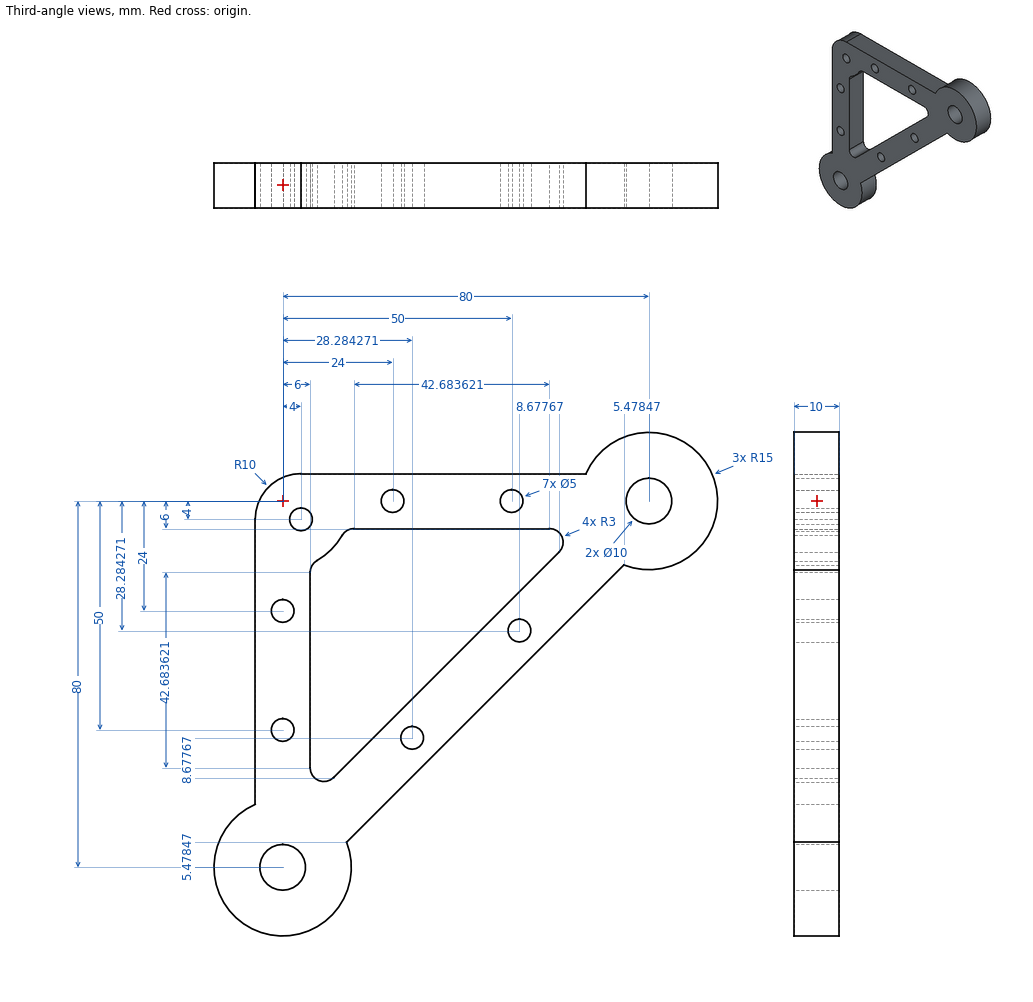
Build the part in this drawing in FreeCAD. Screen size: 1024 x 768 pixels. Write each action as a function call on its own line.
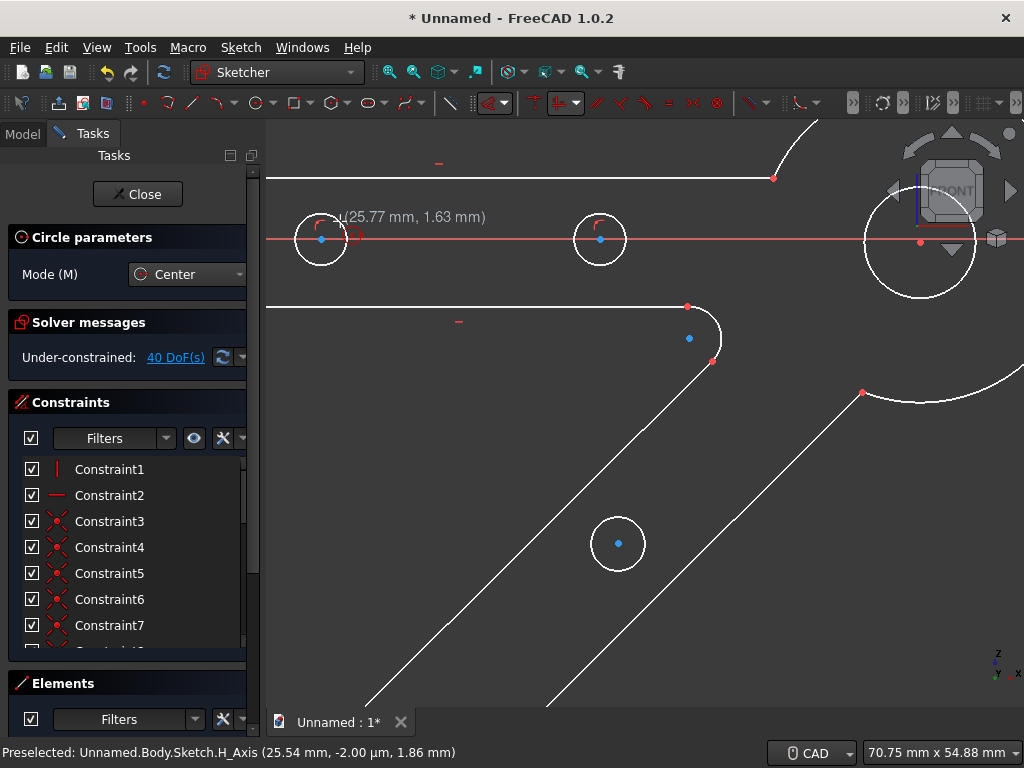
scroll(601, 240, down, 5)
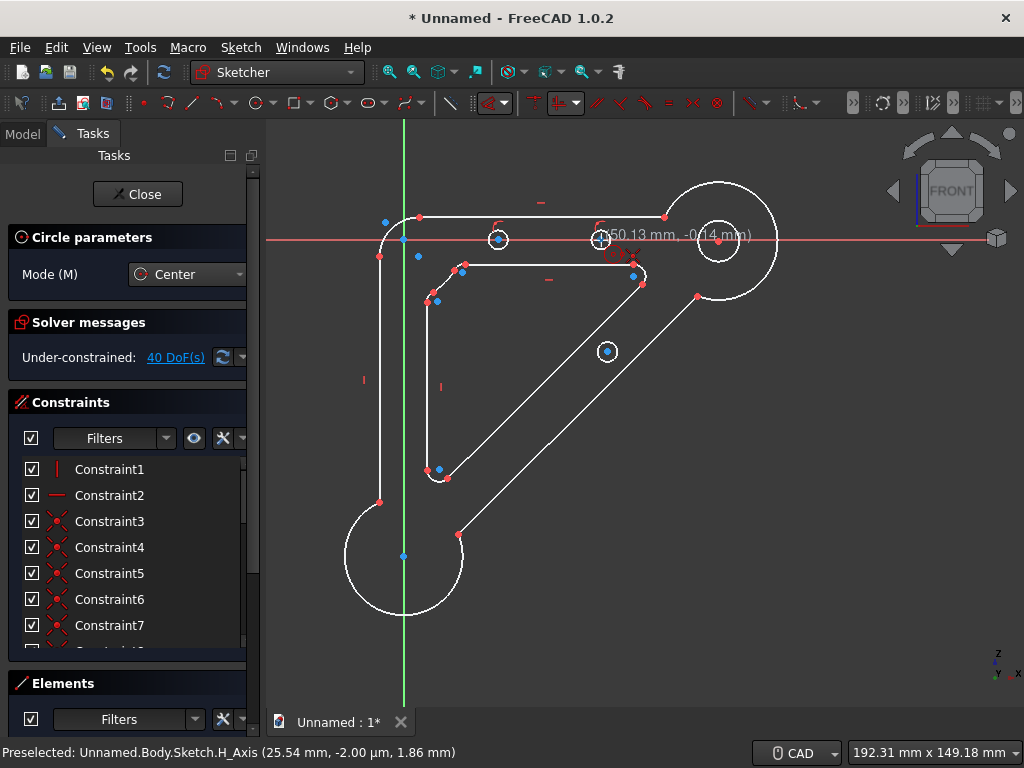
scroll(419, 256, up, 5)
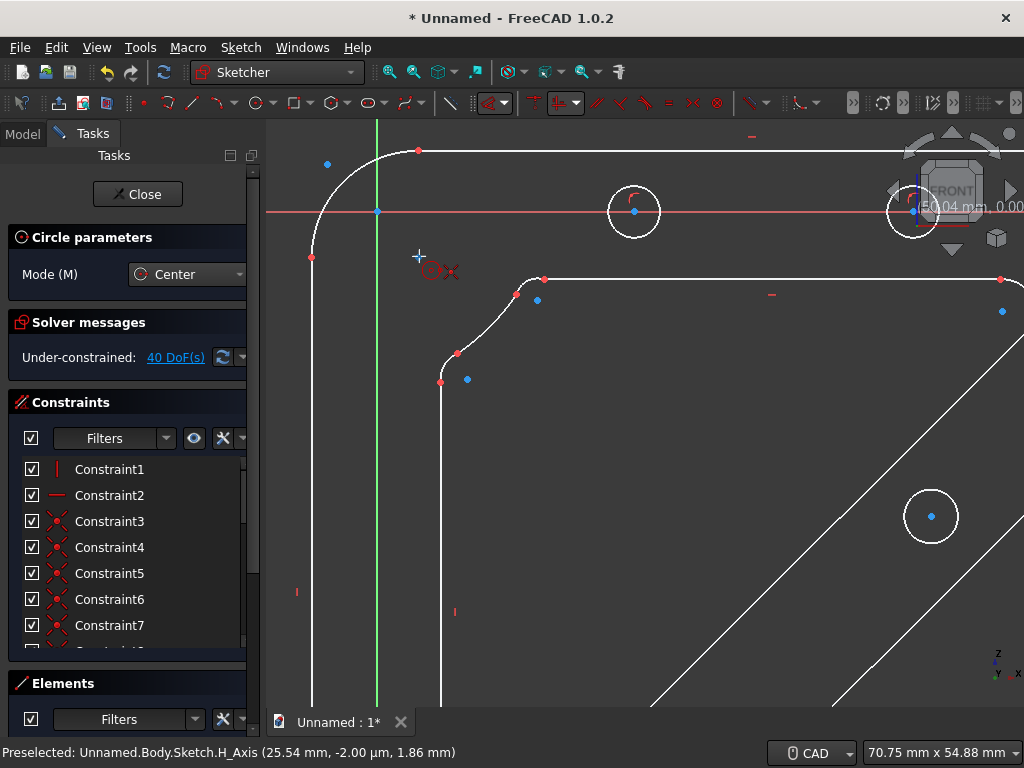
click(420, 255)
click(439, 236)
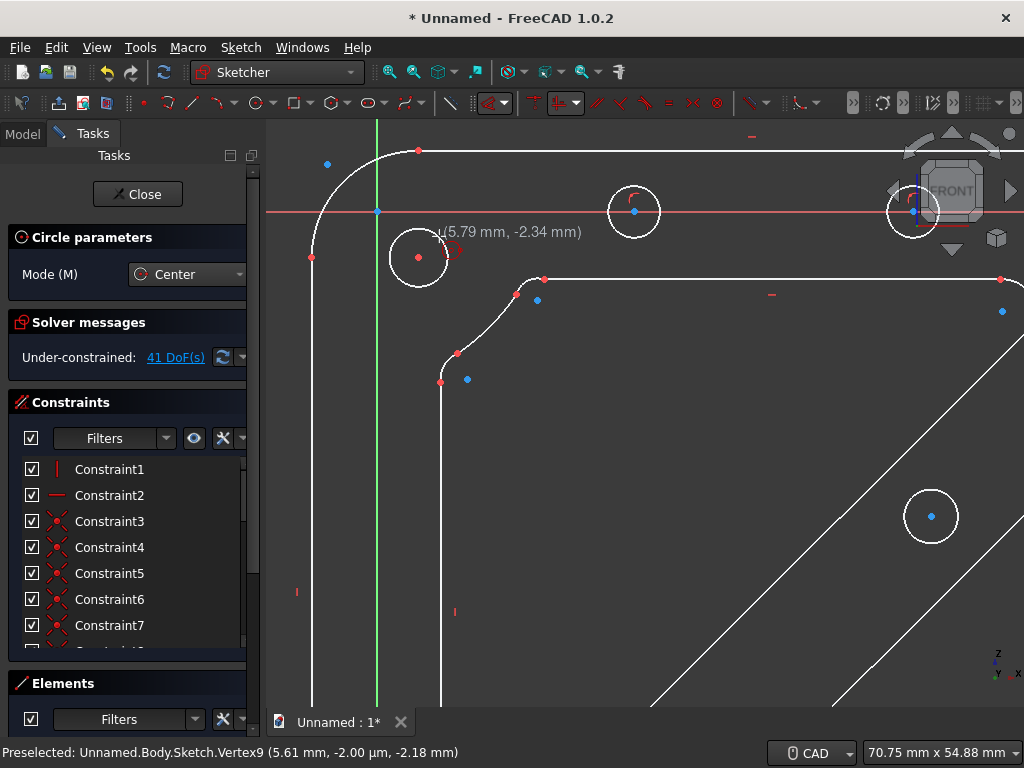
click(377, 469)
click(396, 450)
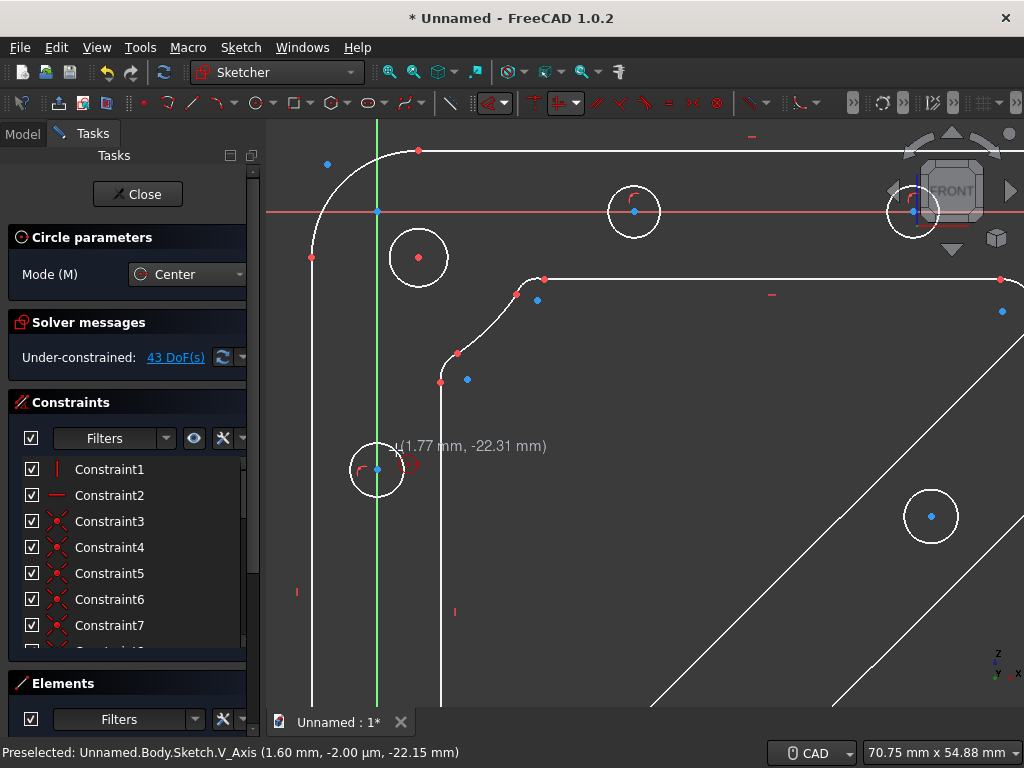
scroll(419, 256, down, 5)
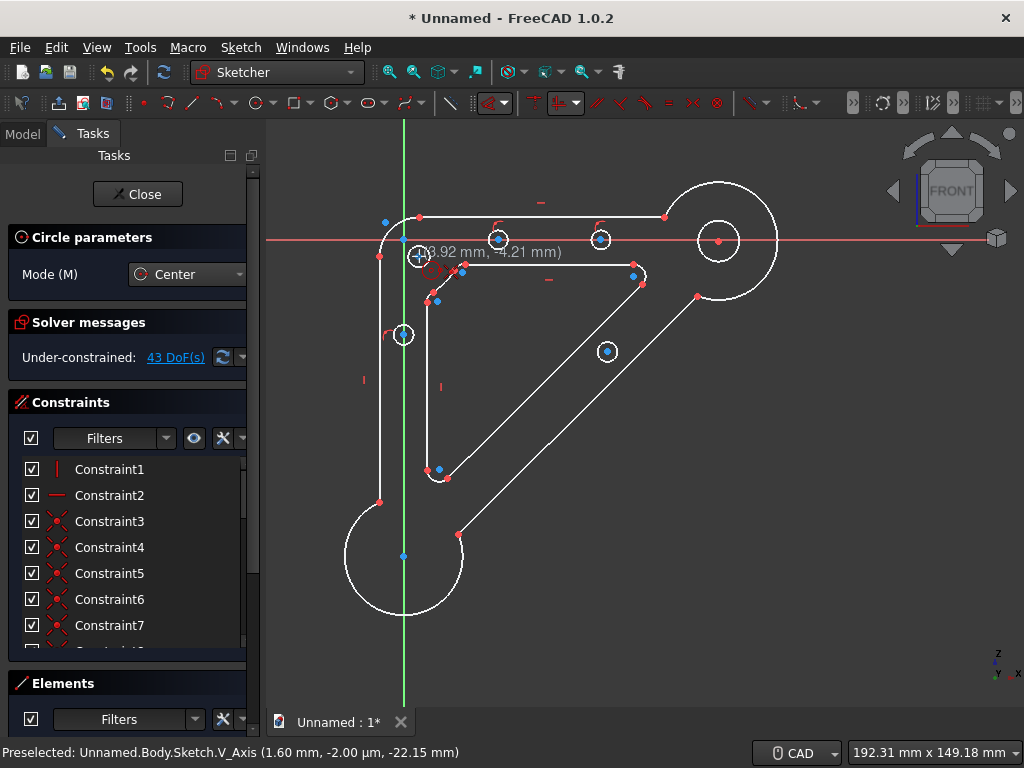
scroll(515, 444, up, 5)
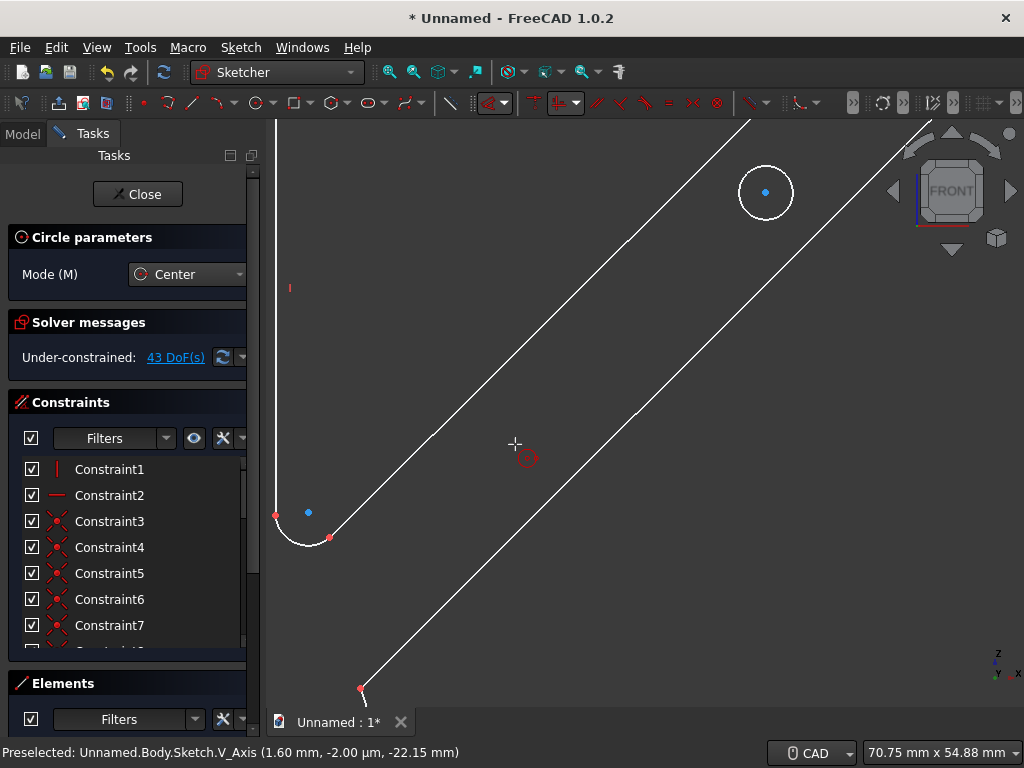
click(515, 442)
click(534, 423)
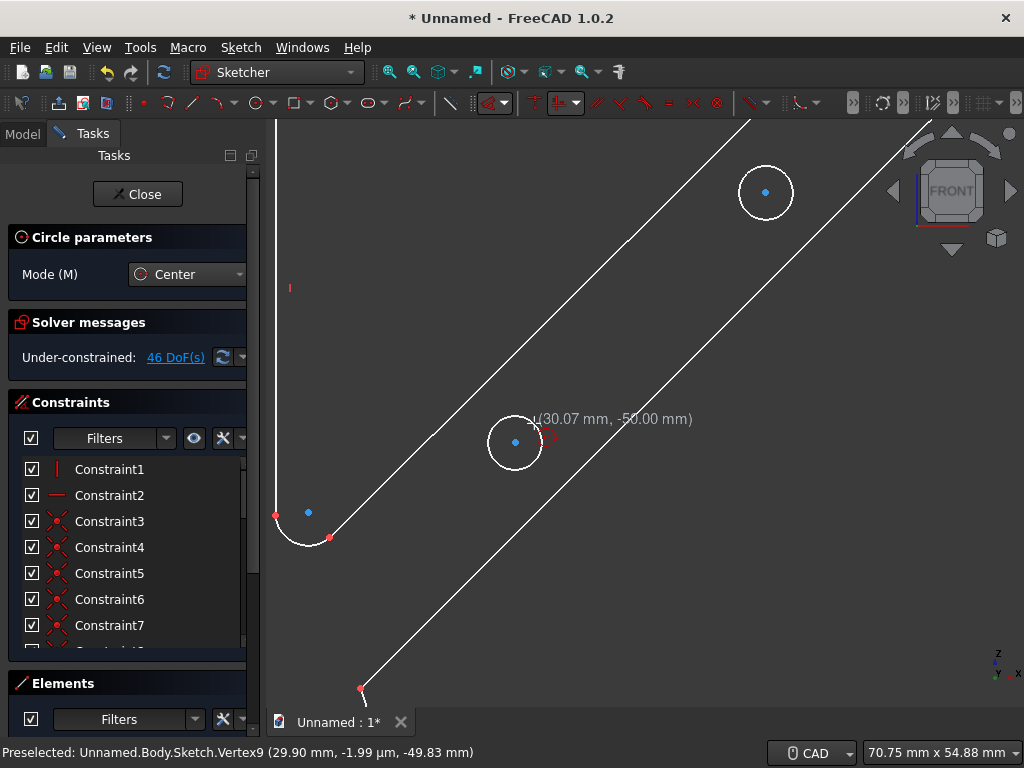
scroll(515, 444, down, 5)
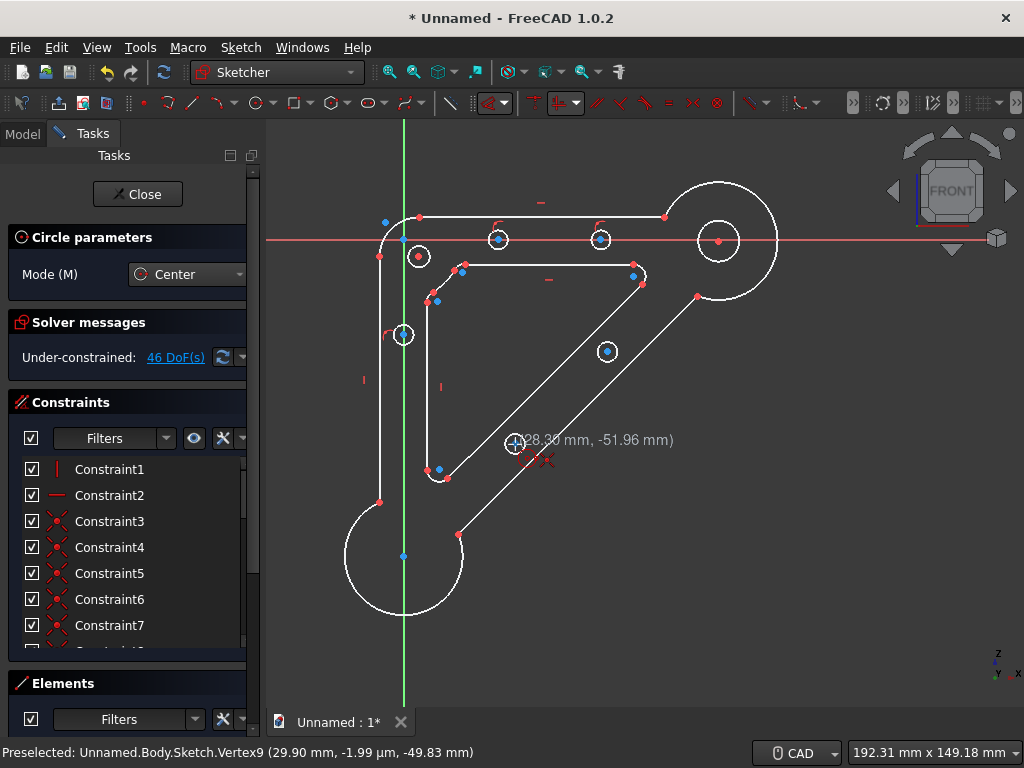
scroll(404, 437, up, 5)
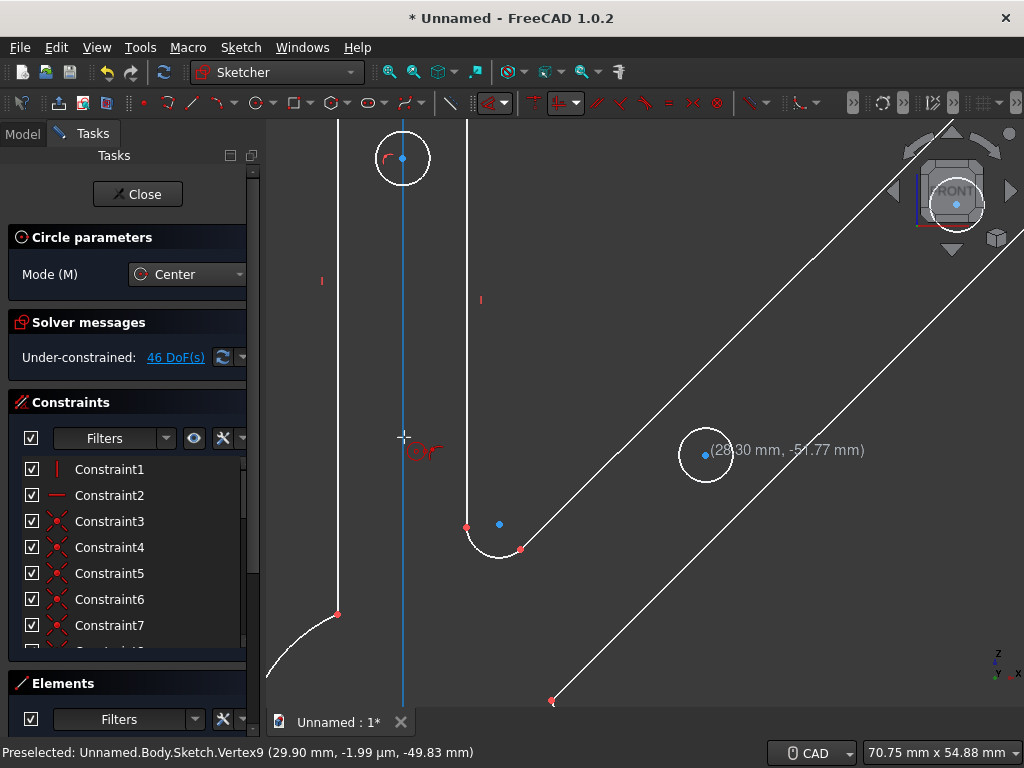
click(403, 436)
click(422, 417)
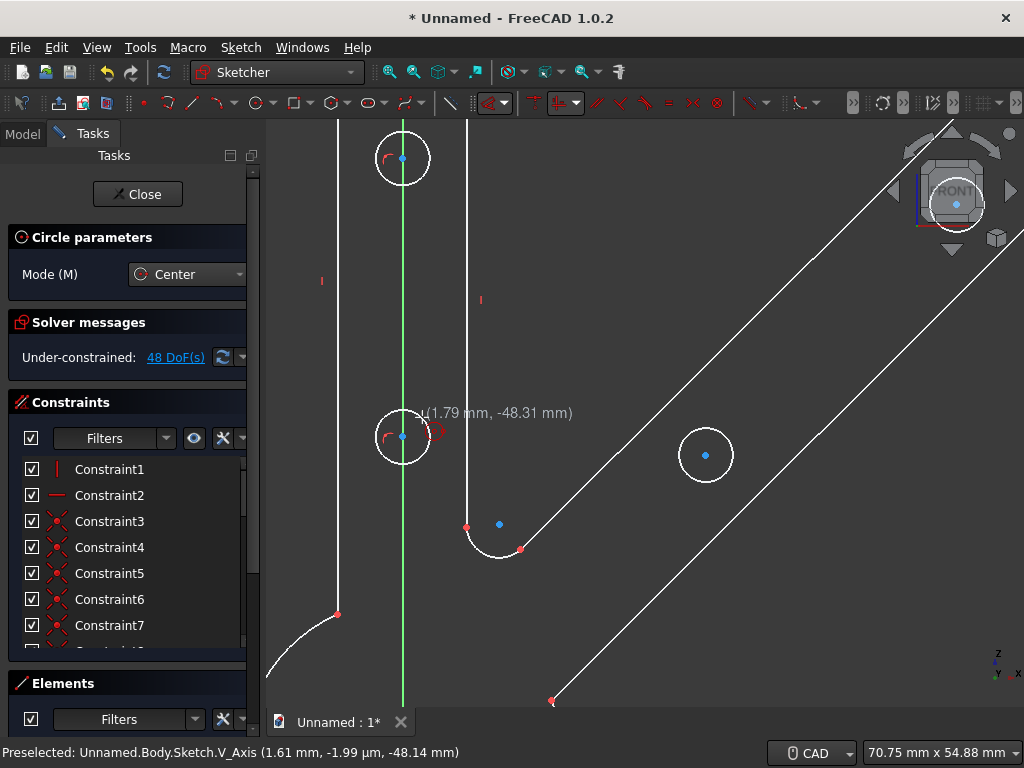
scroll(404, 437, down, 5)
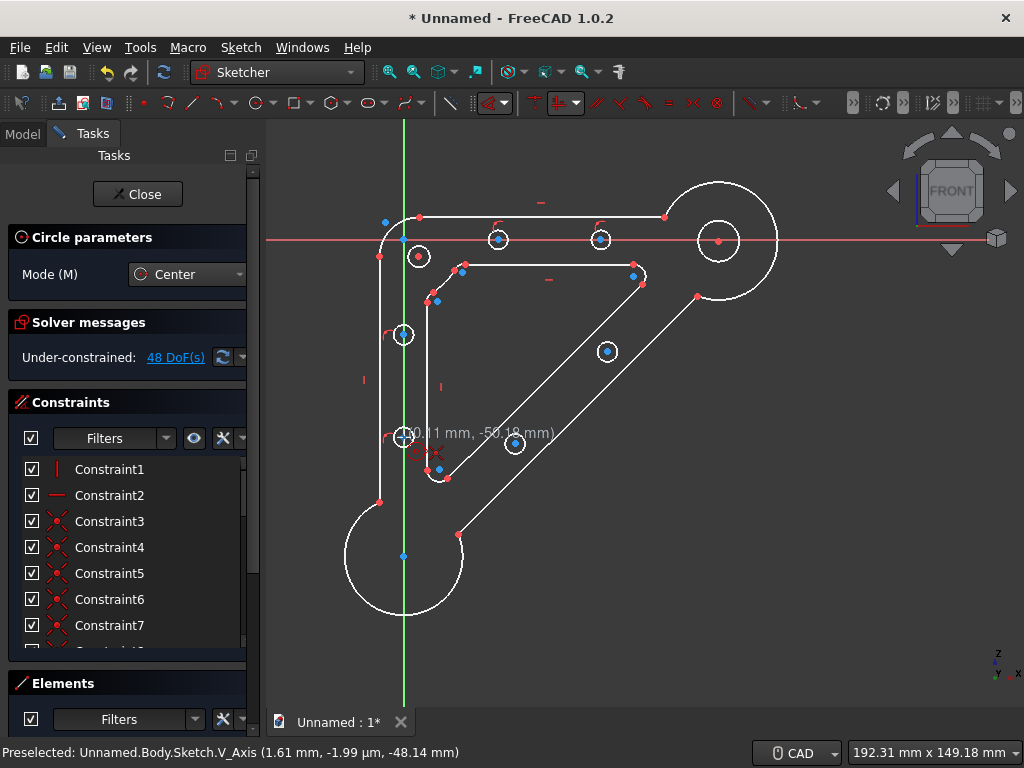
click(404, 555)
click(422, 549)
key(Escape)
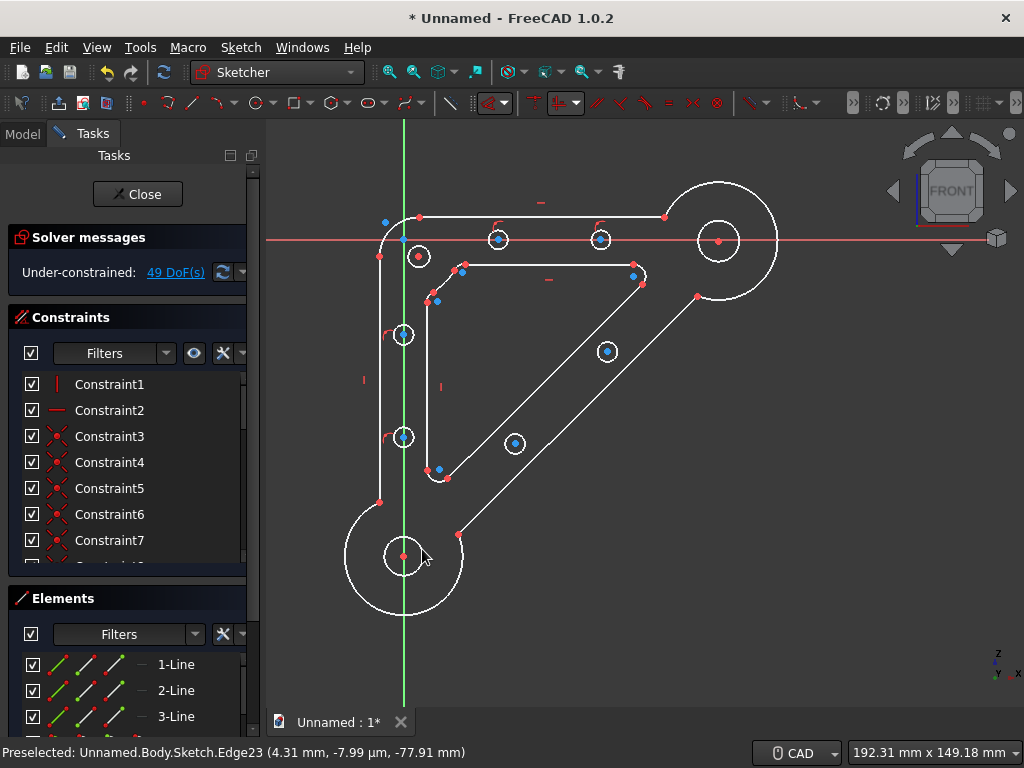
click(380, 429)